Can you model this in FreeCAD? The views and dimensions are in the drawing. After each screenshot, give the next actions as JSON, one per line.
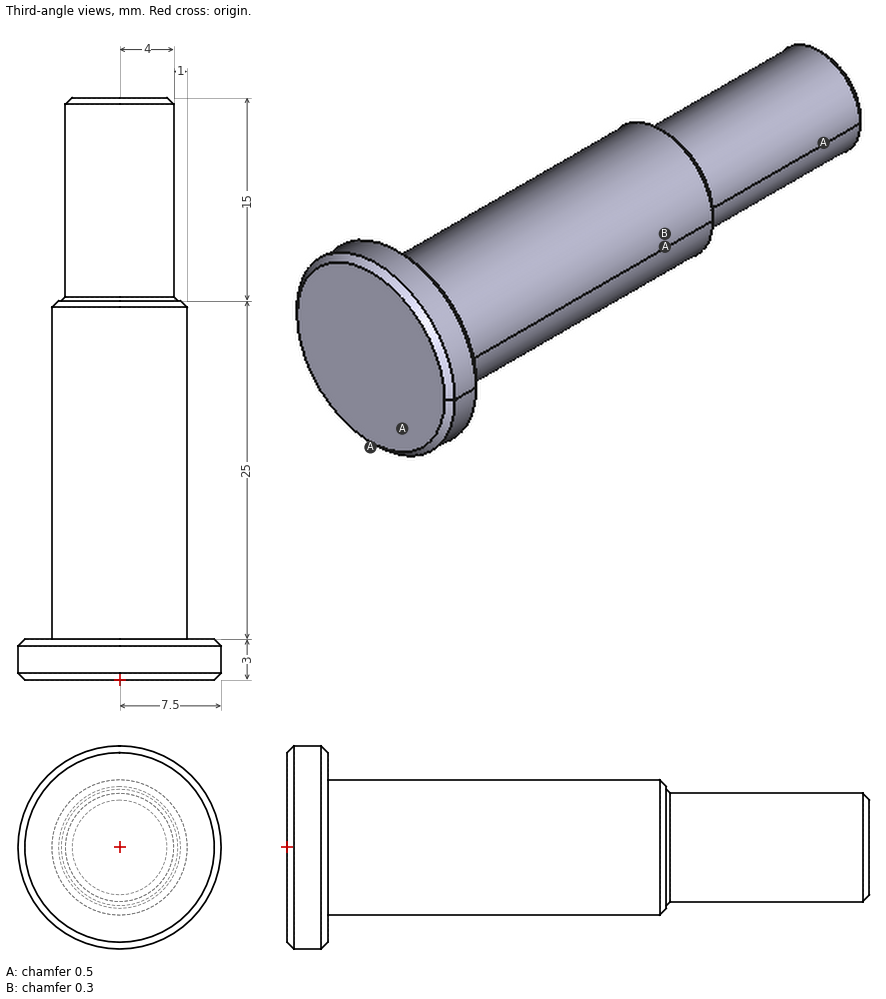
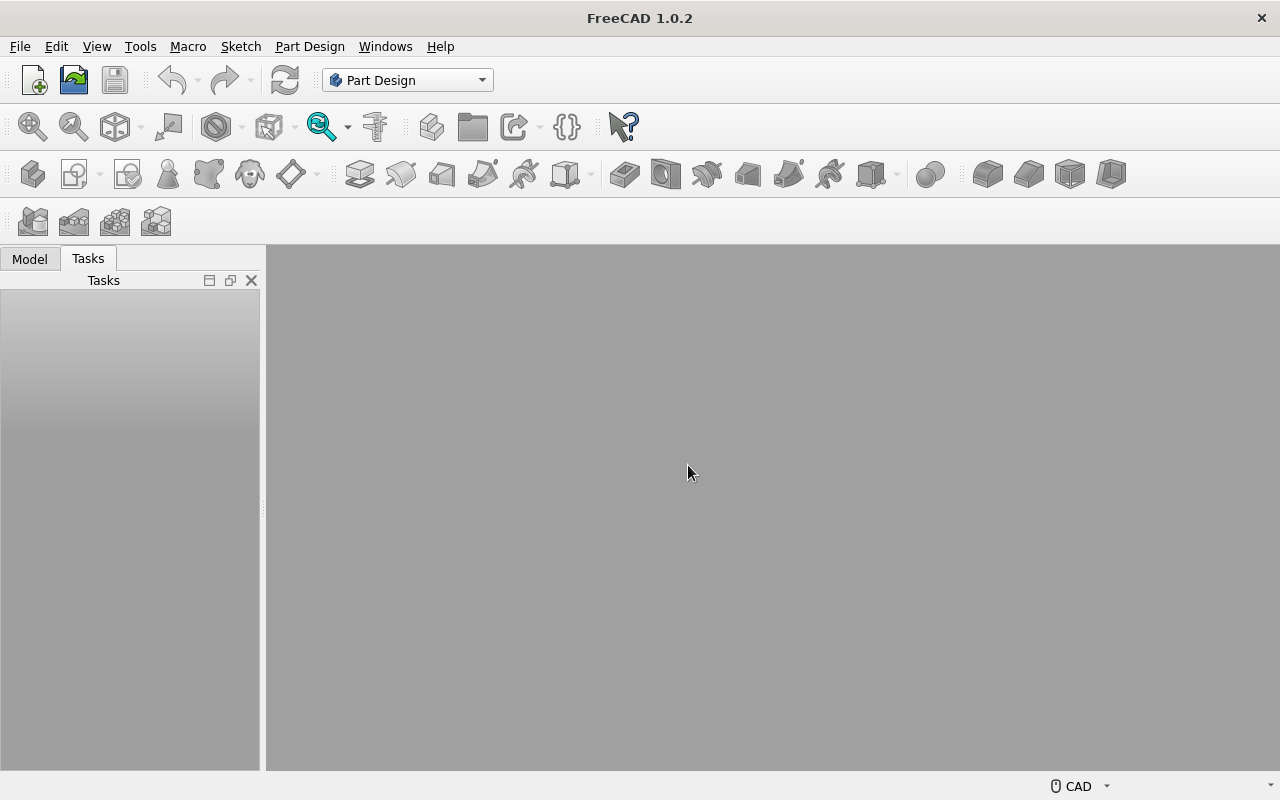
{"action": "left_click", "coordinate": [33, 80]}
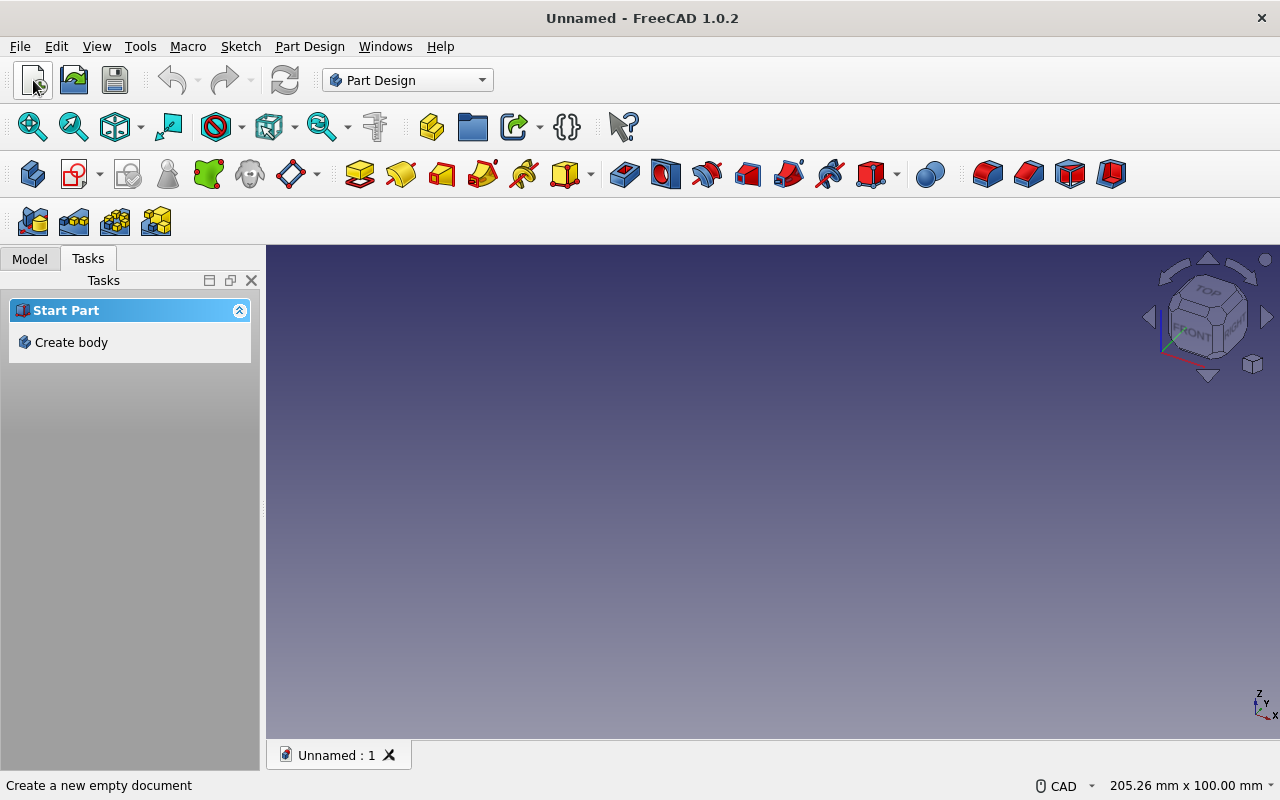
{"action": "left_click", "coordinate": [74, 174]}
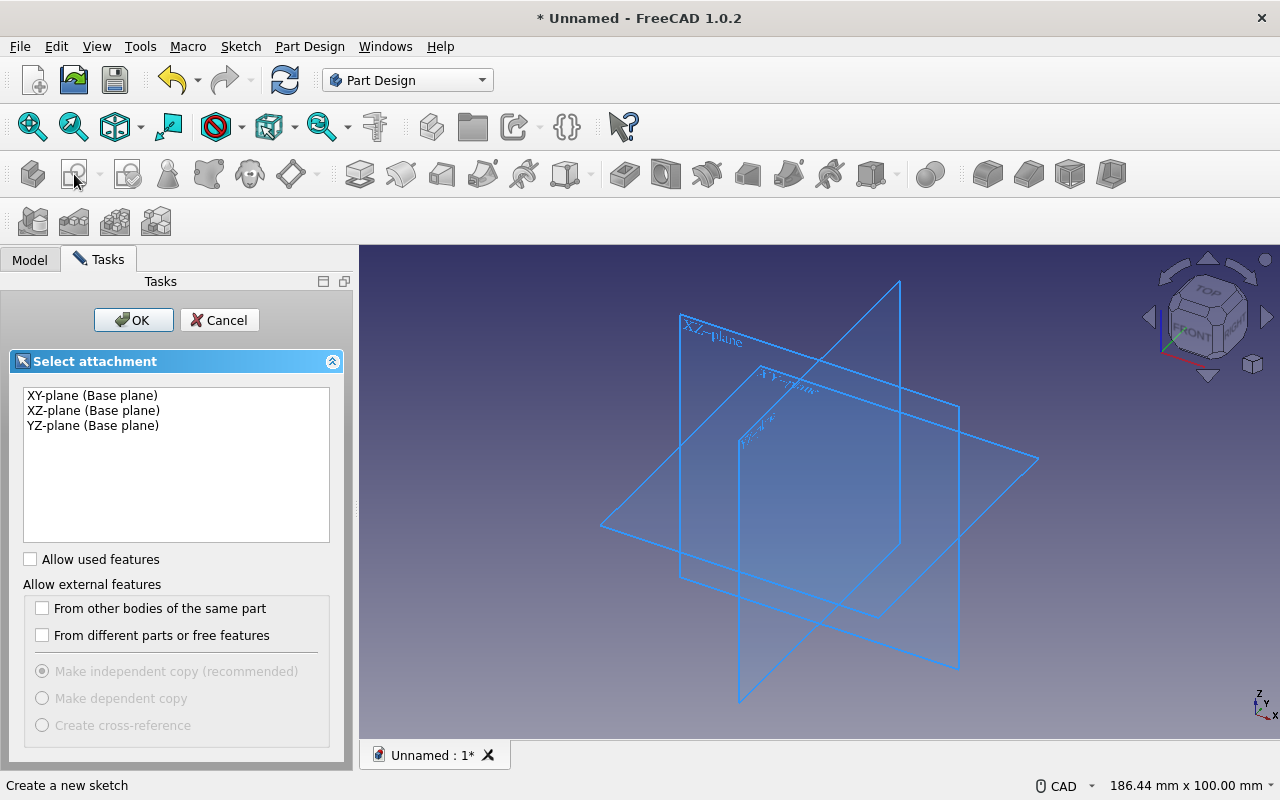
{"action": "left_click", "coordinate": [84, 396]}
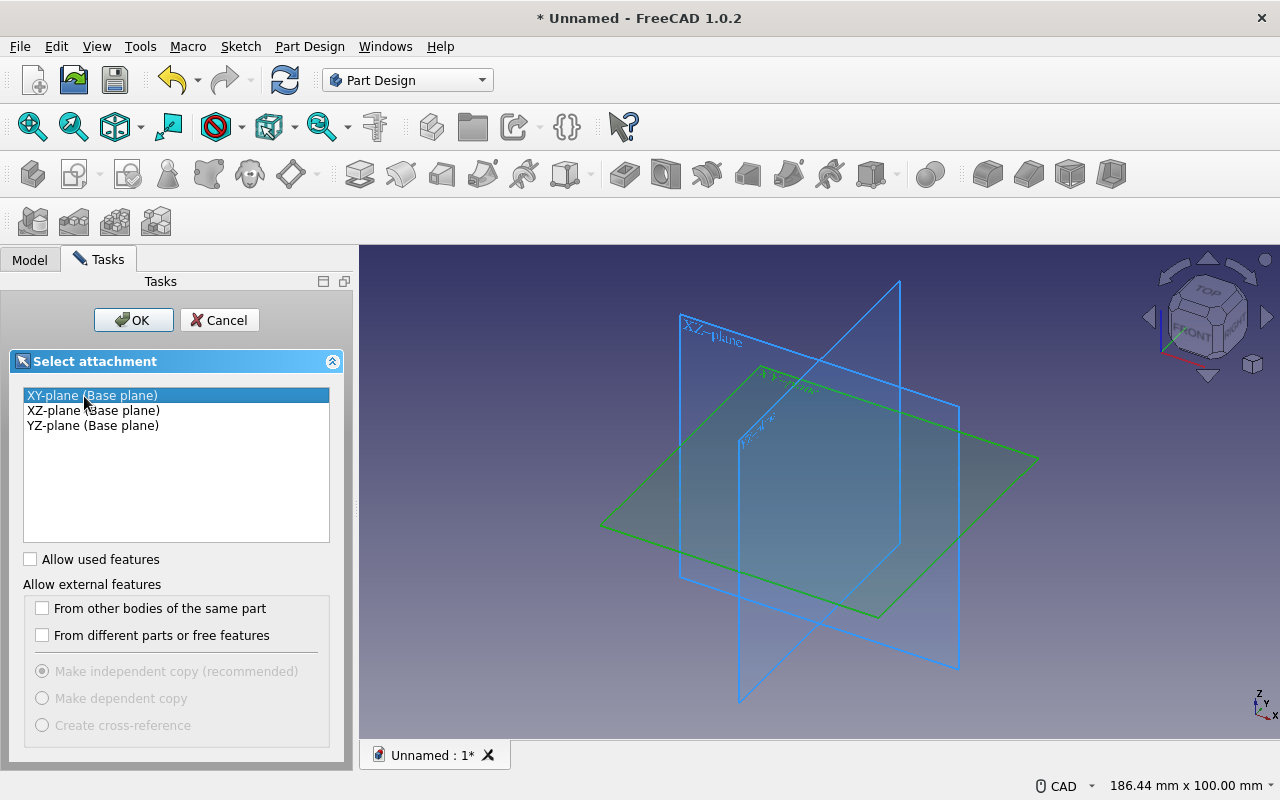
{"action": "left_click", "coordinate": [134, 320]}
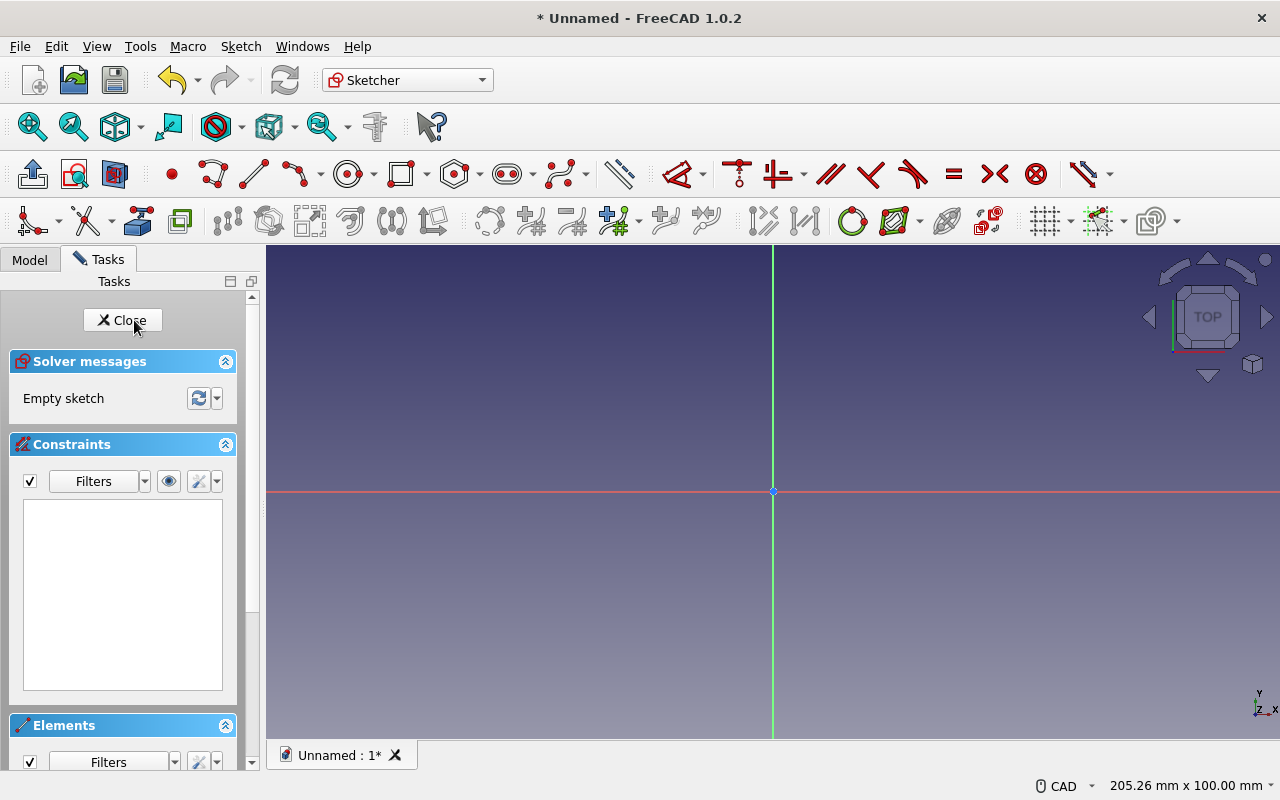
{"action": "scroll", "coordinate": [311, 711], "scroll_direction": "down", "scroll_amount": 1}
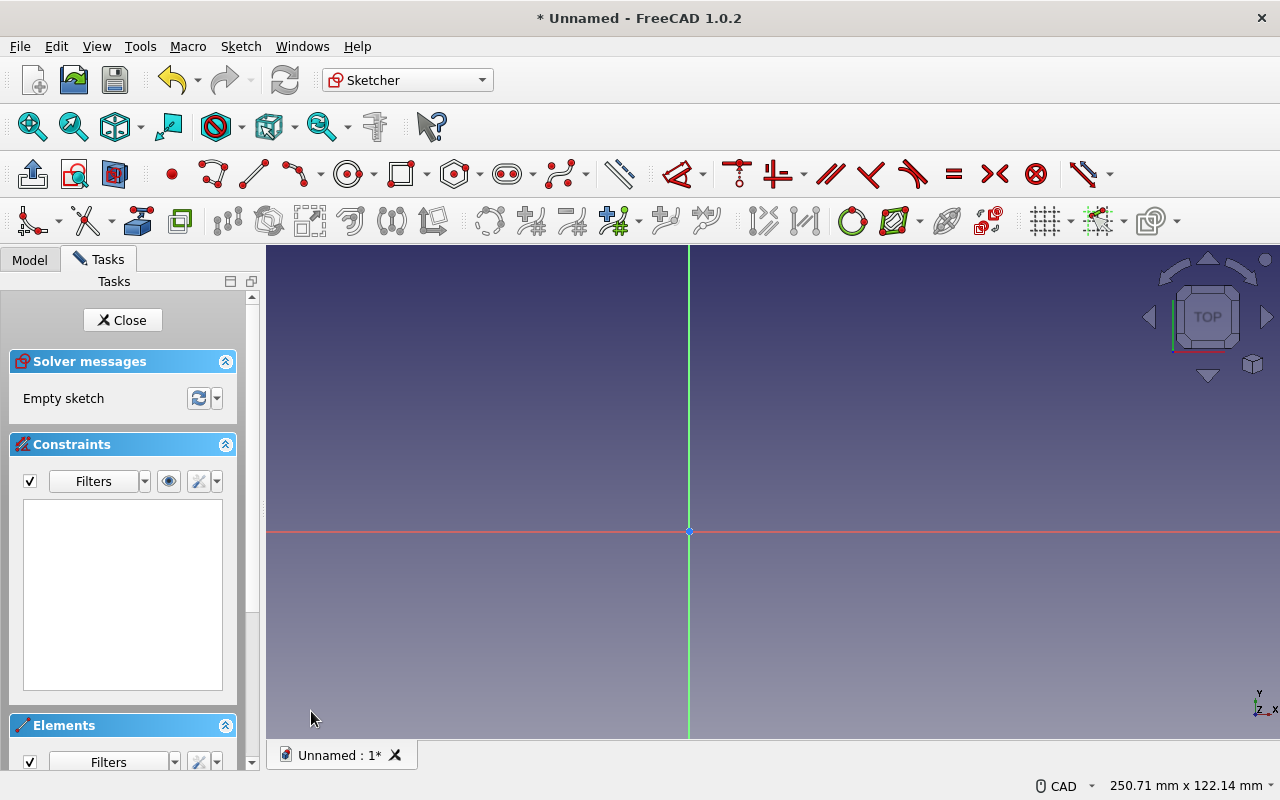
{"action": "scroll", "coordinate": [704, 388], "scroll_direction": "up", "scroll_amount": 3}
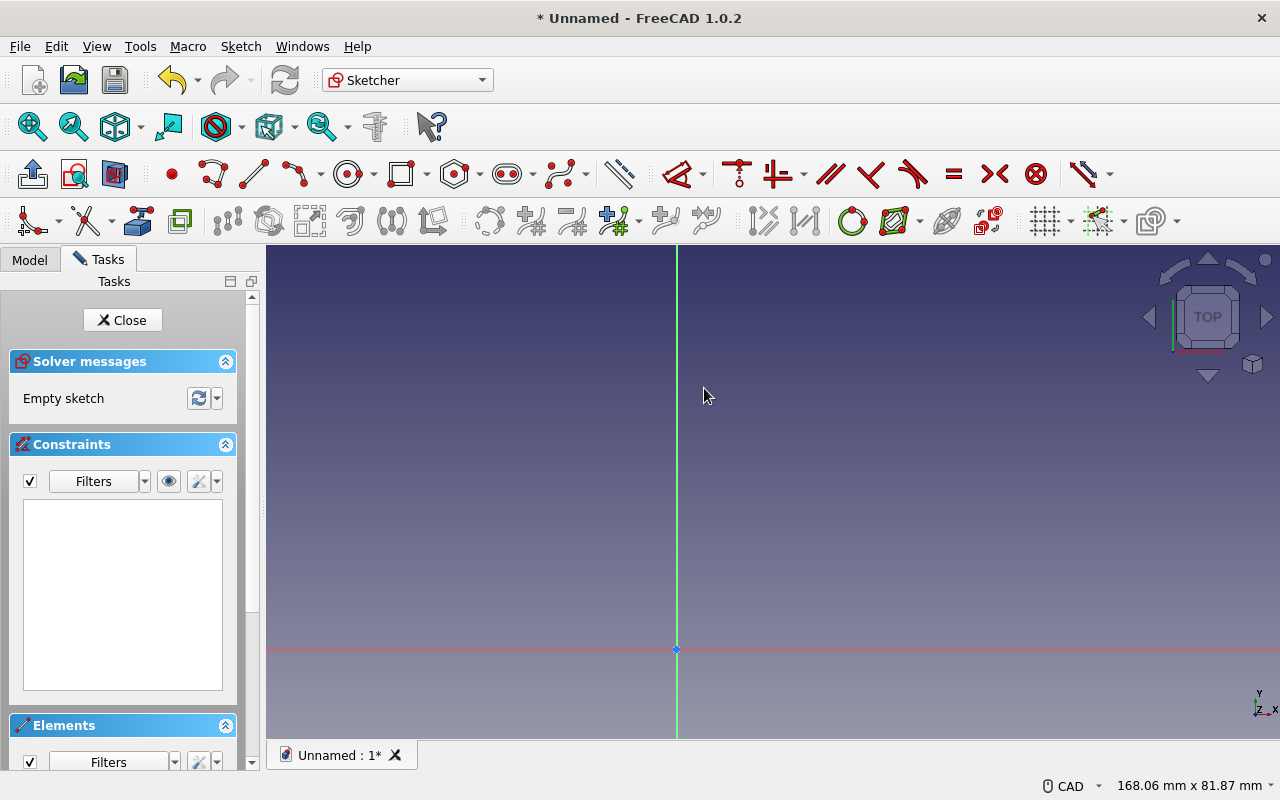
{"action": "left_click", "coordinate": [213, 174]}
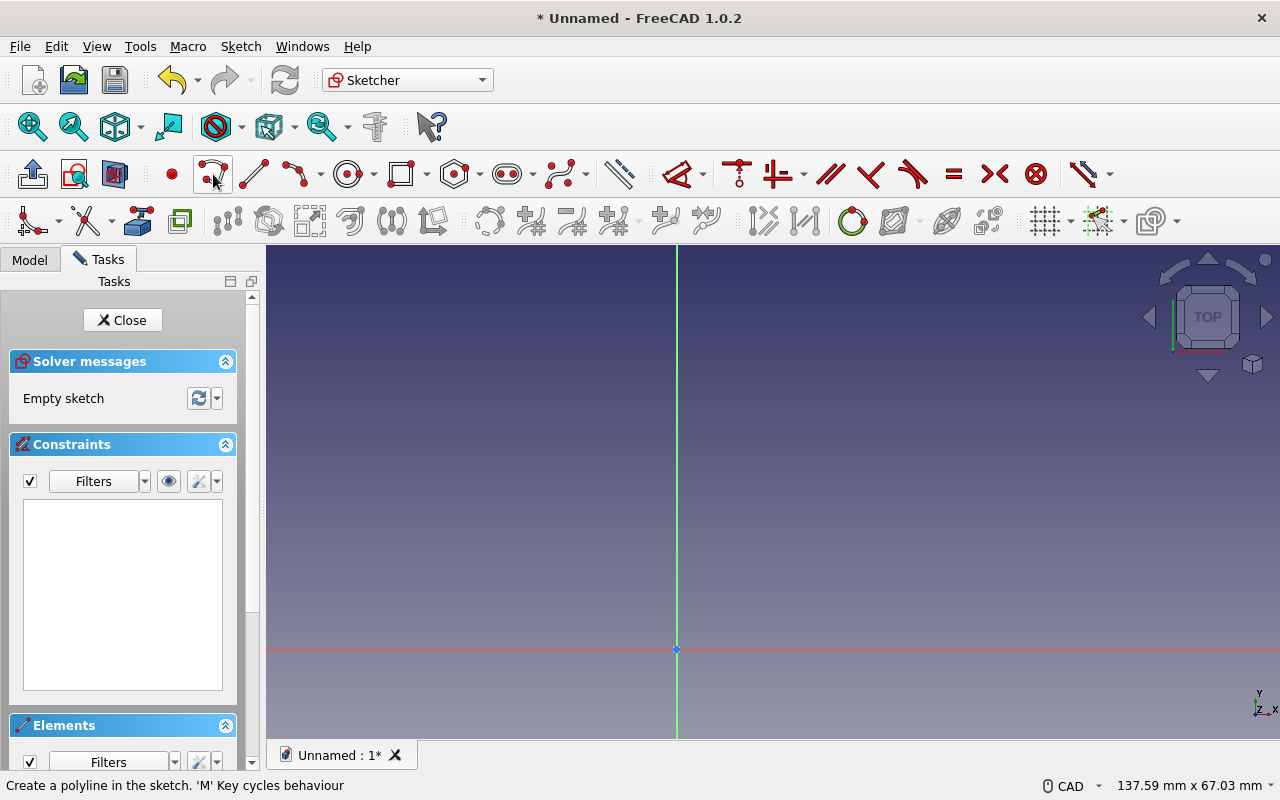
{"action": "left_click", "coordinate": [677, 650]}
{"action": "left_click", "coordinate": [732, 641]}
{"action": "left_click", "coordinate": [732, 628]}
{"action": "left_click", "coordinate": [714, 628]}
{"action": "left_click", "coordinate": [714, 444]}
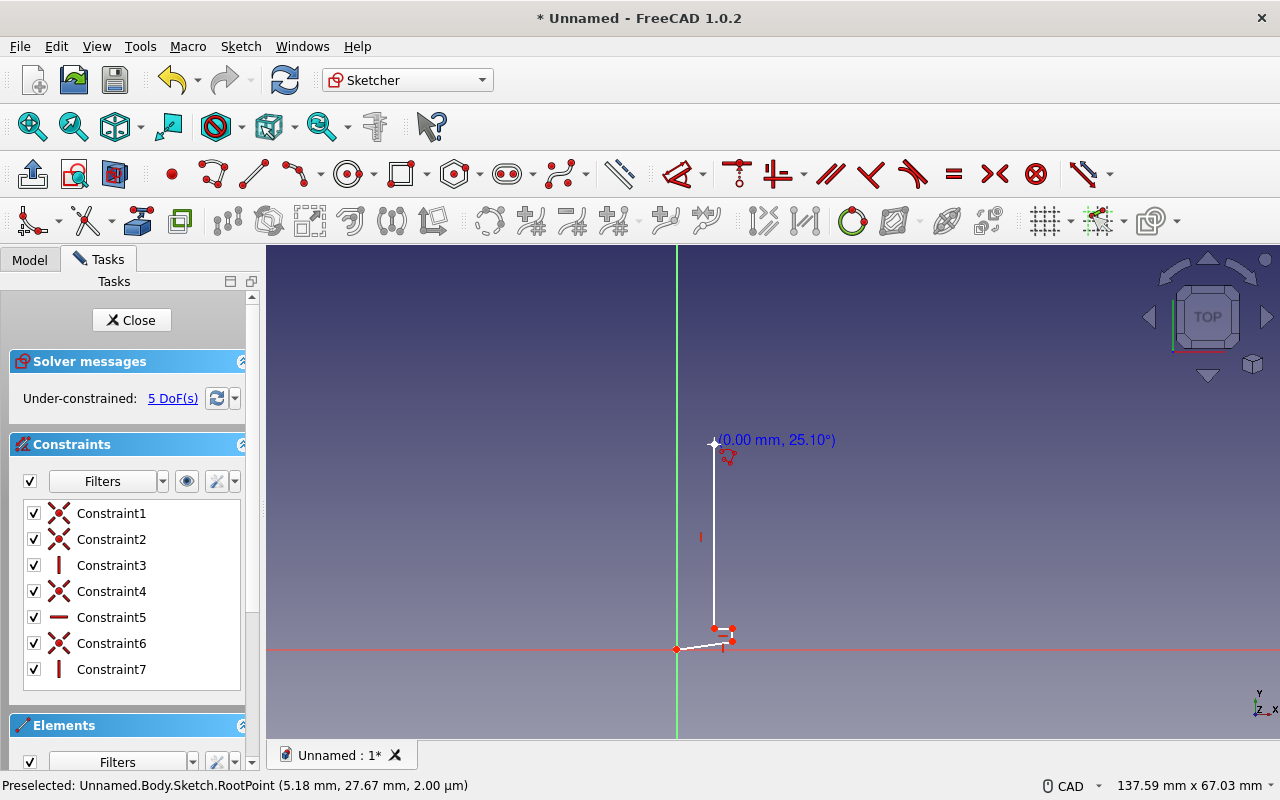
{"action": "scroll", "coordinate": [706, 444], "scroll_direction": "up", "scroll_amount": 4}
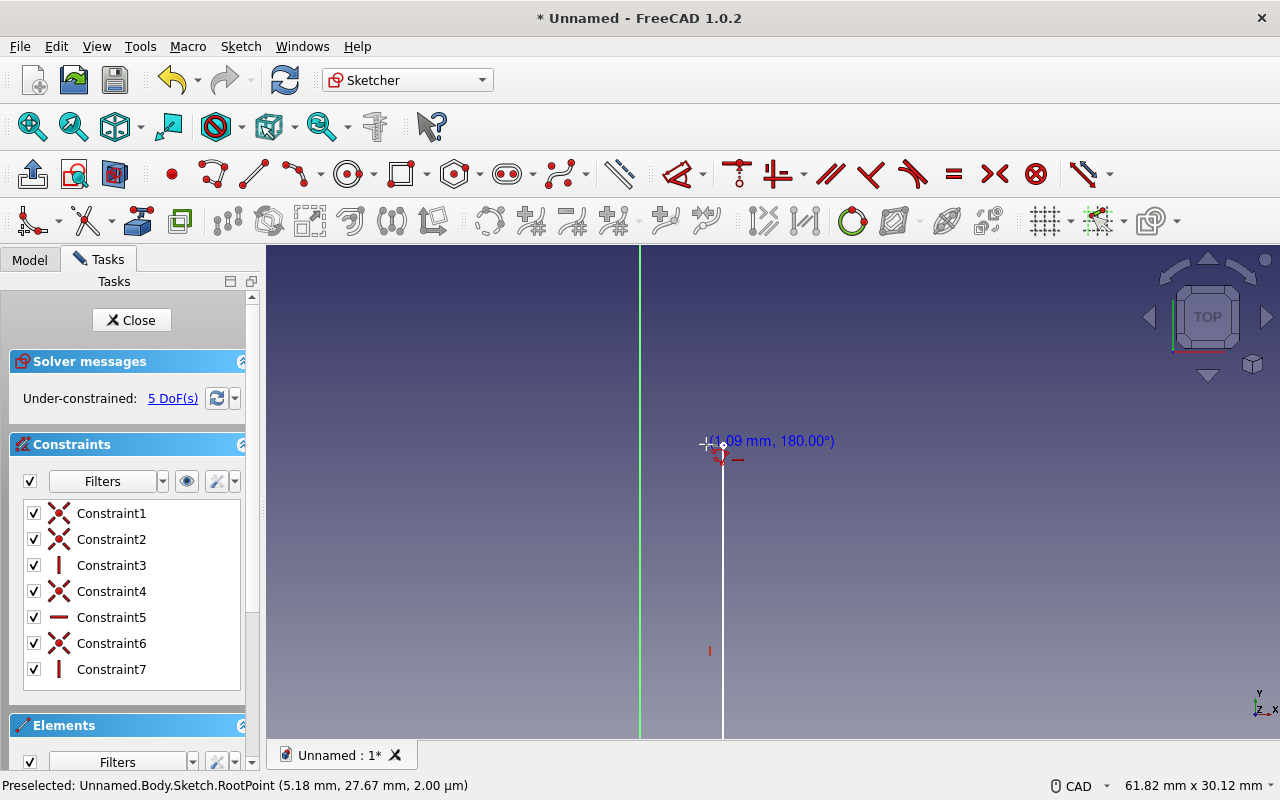
{"action": "left_click", "coordinate": [706, 444]}